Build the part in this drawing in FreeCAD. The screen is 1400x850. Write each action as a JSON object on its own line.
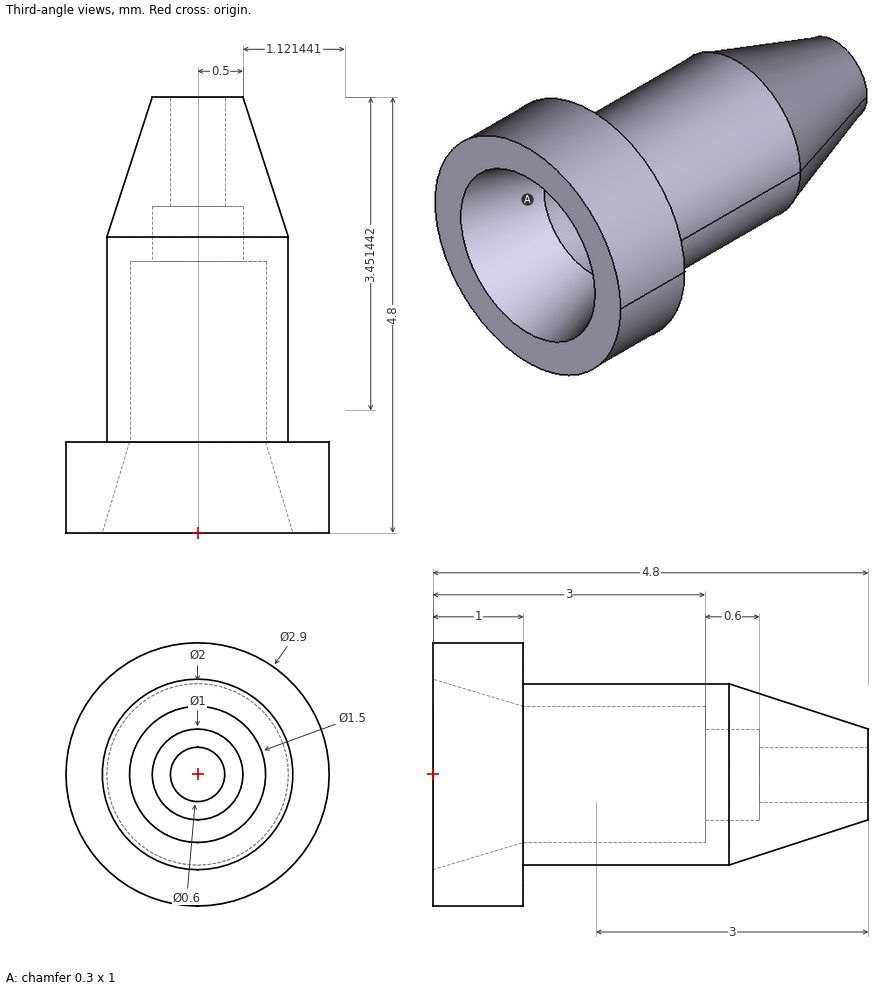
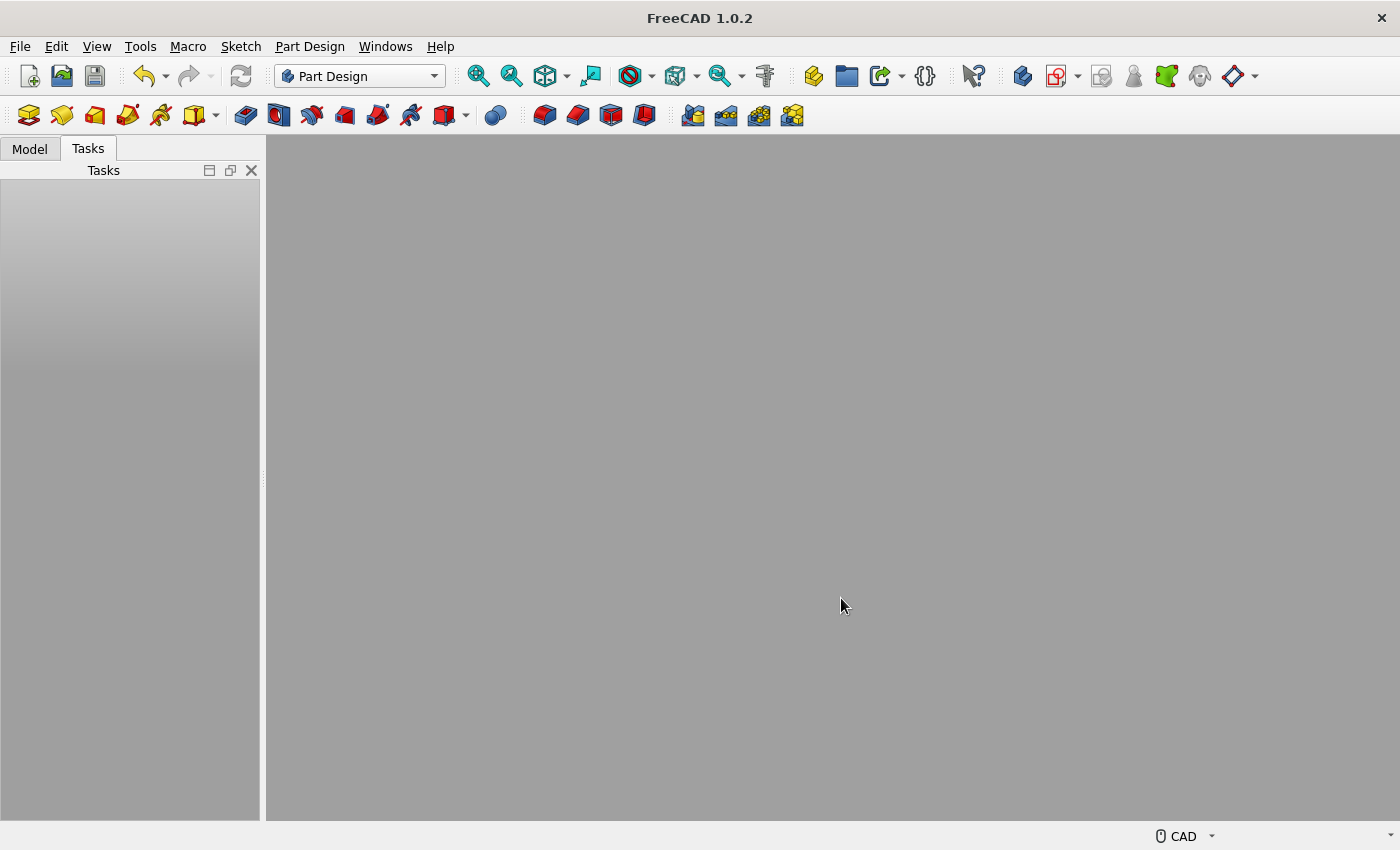
{"action": "left_click", "coordinate": [29, 76]}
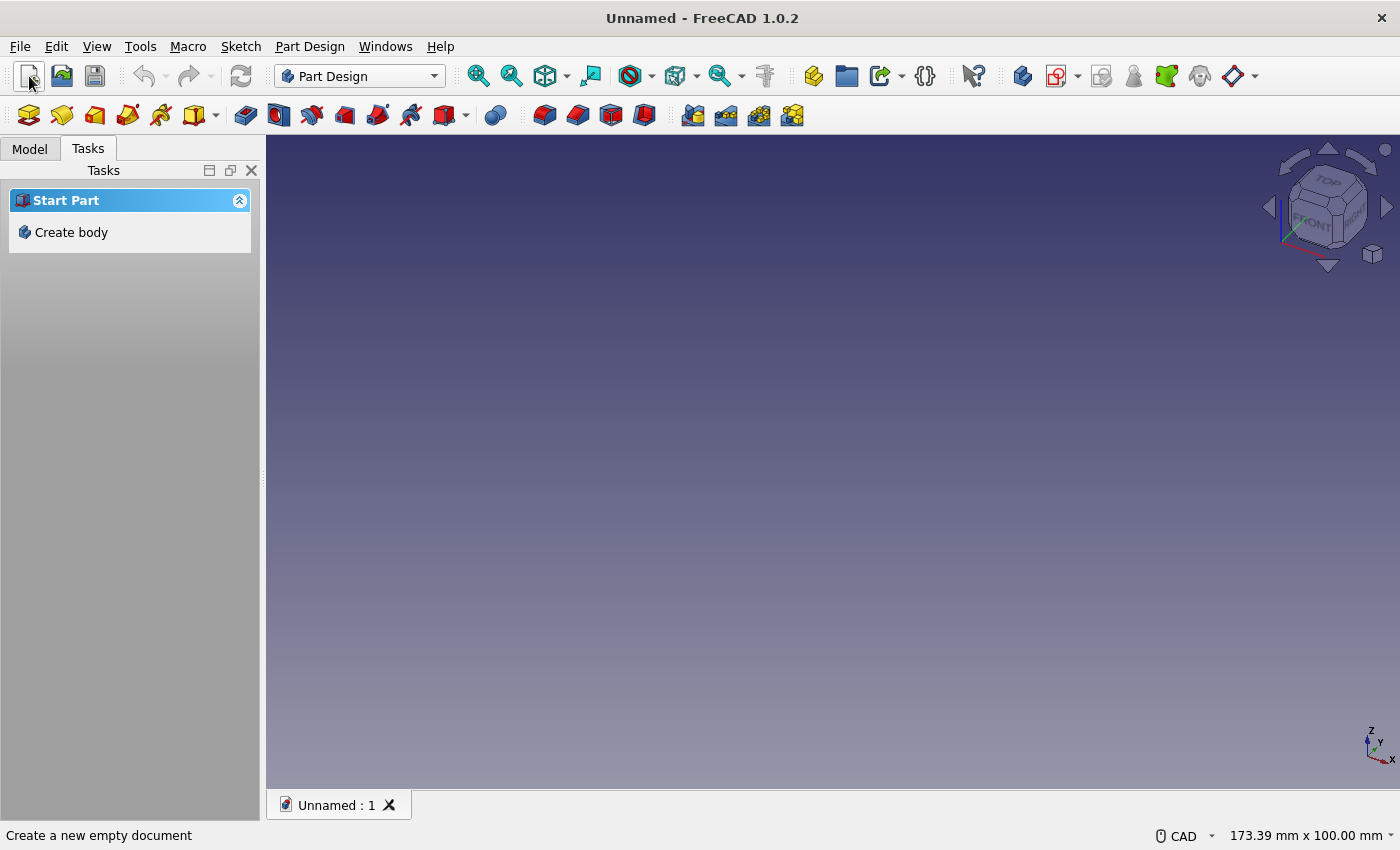
{"action": "left_click", "coordinate": [1056, 76]}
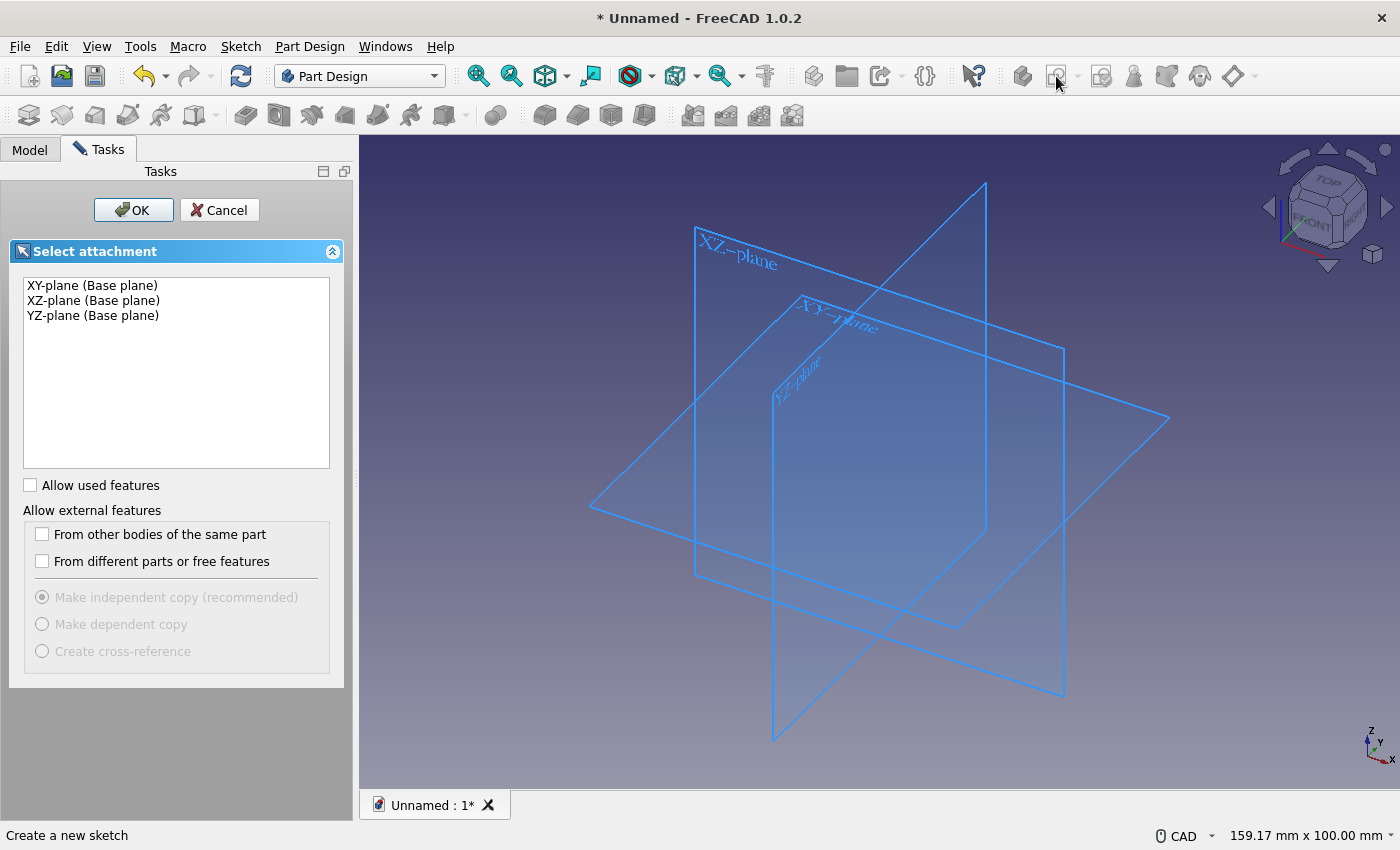
{"action": "left_click", "coordinate": [84, 300]}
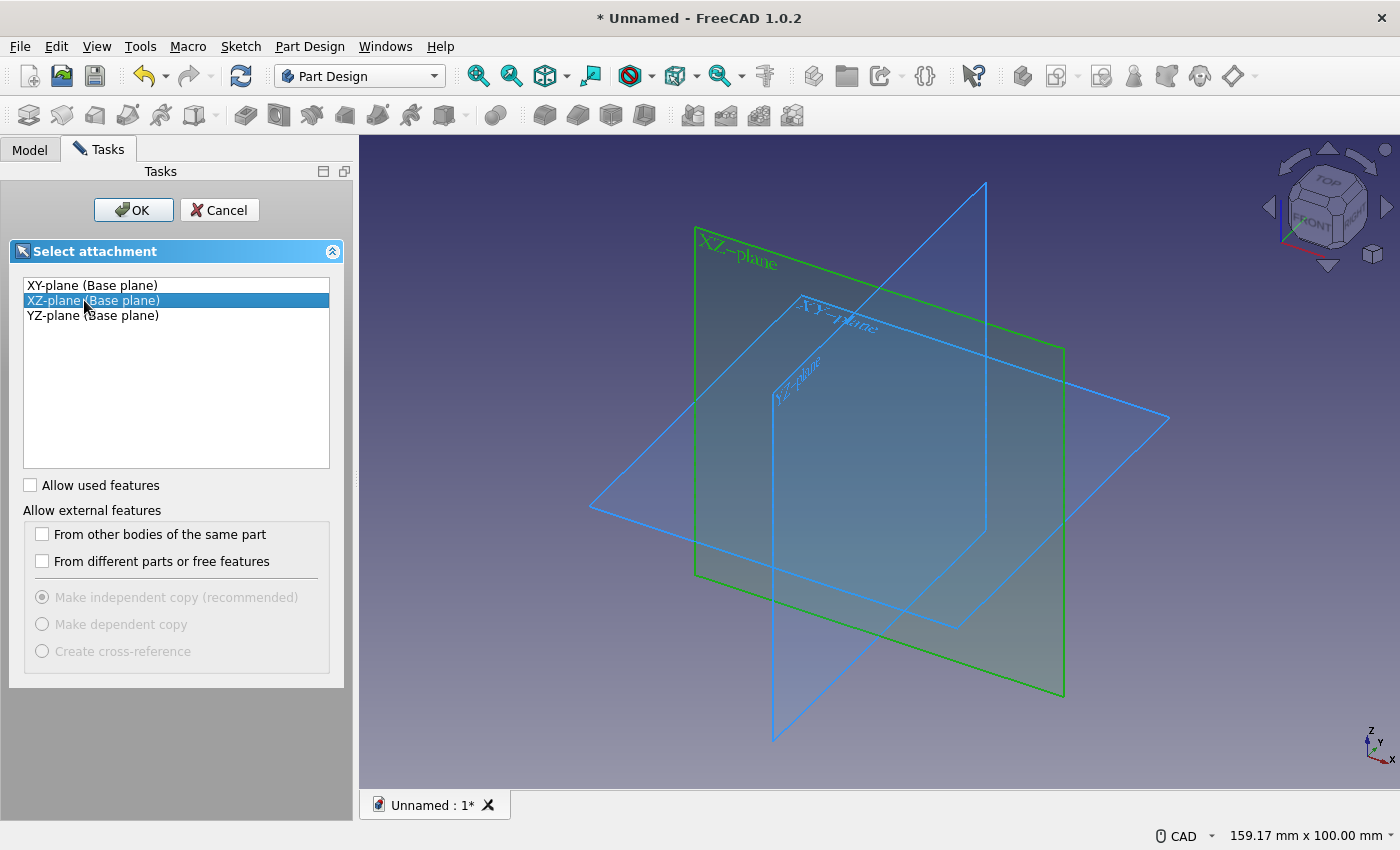
{"action": "left_click", "coordinate": [134, 210]}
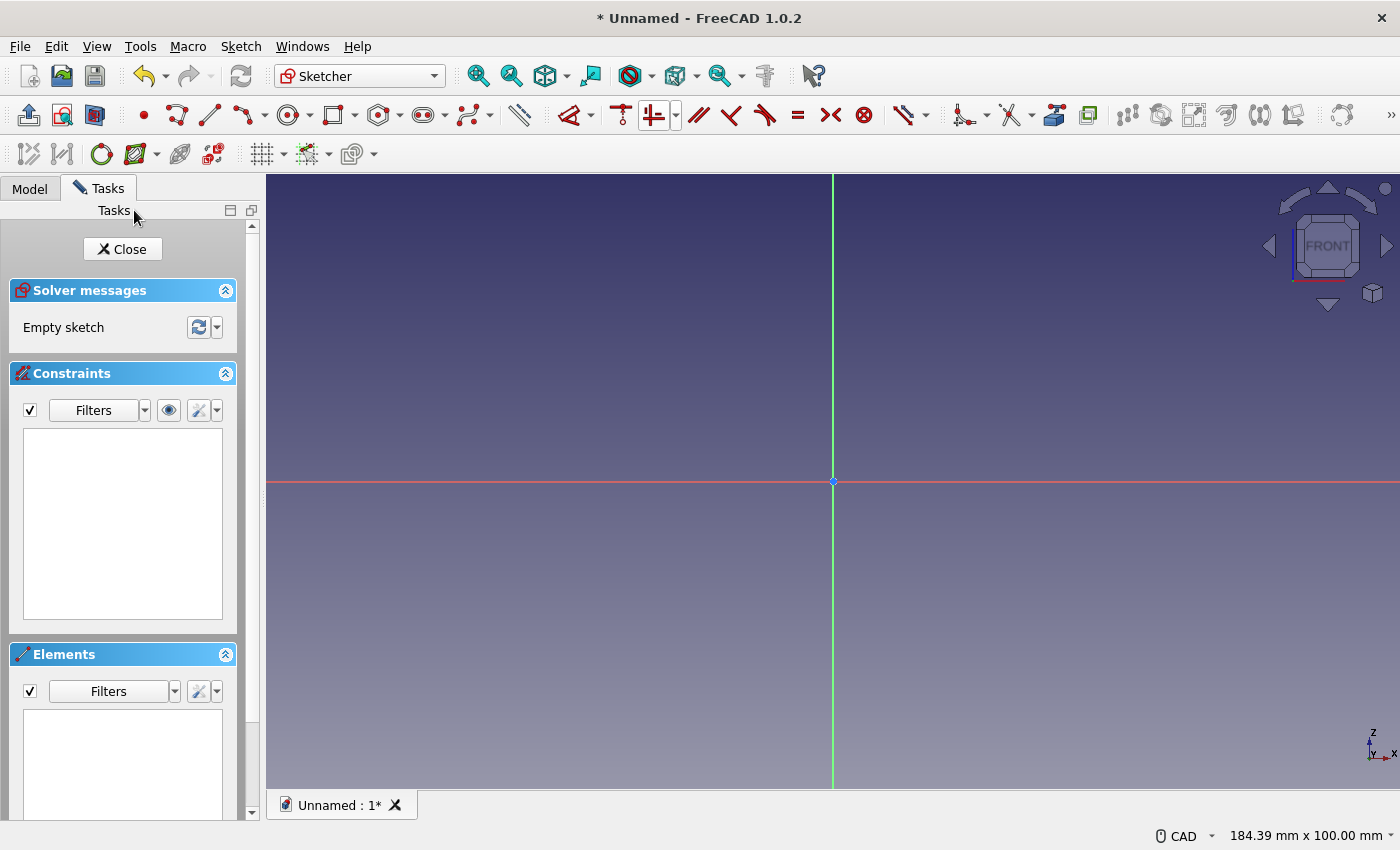
{"action": "scroll", "coordinate": [837, 481], "scroll_direction": "up", "scroll_amount": 15}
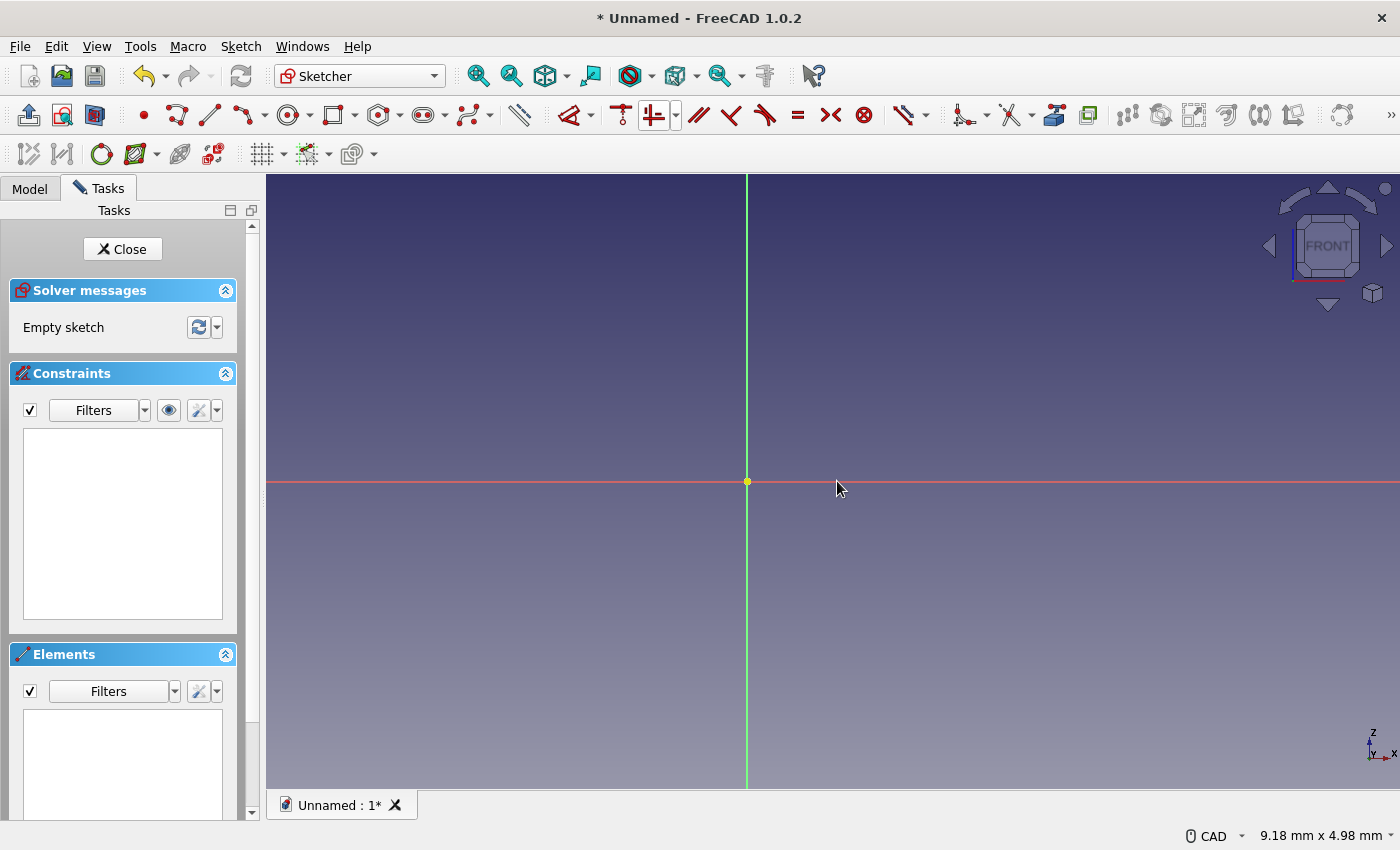
{"action": "scroll", "coordinate": [712, 482], "scroll_direction": "up", "scroll_amount": 2}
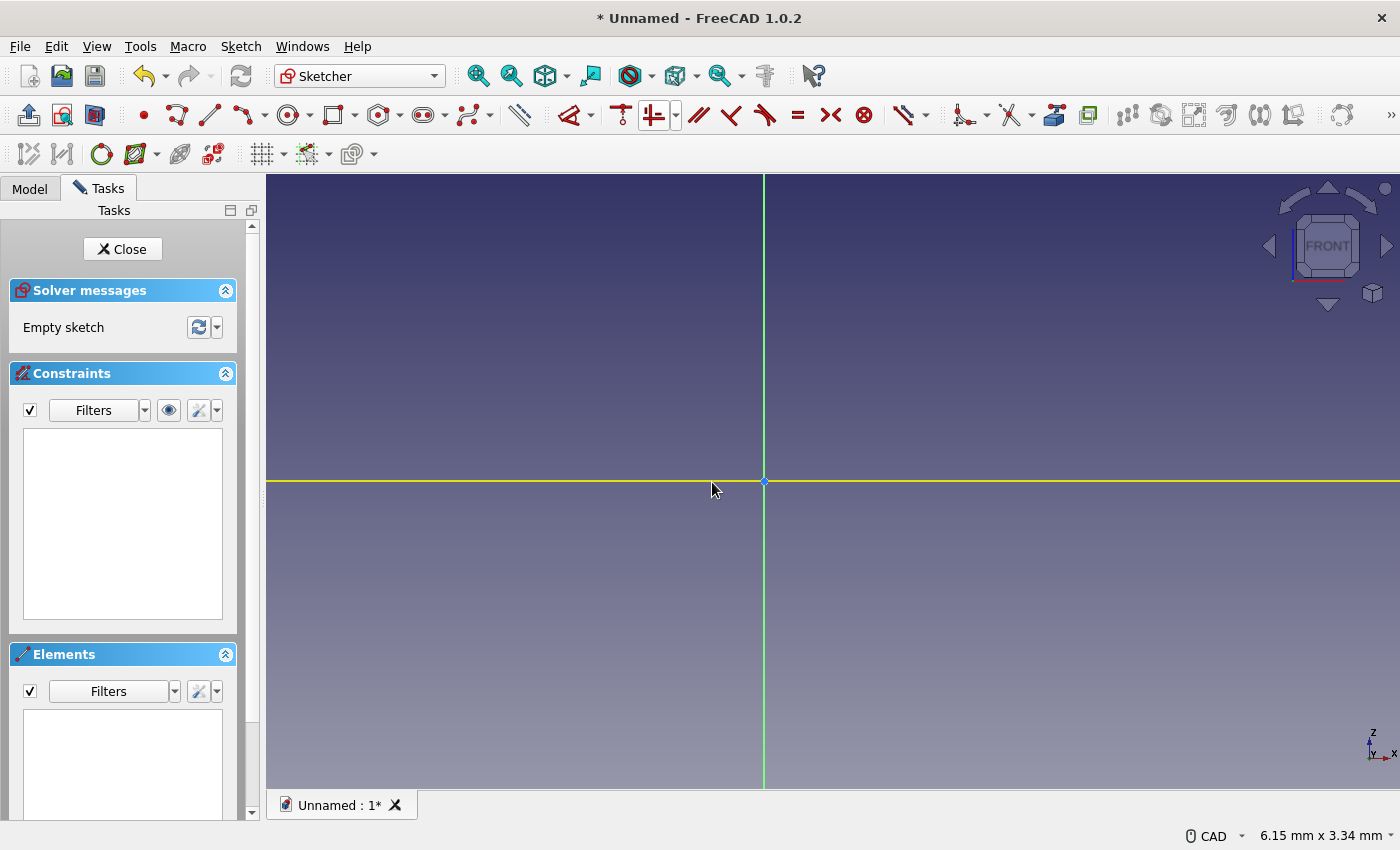
{"action": "left_click", "coordinate": [288, 116]}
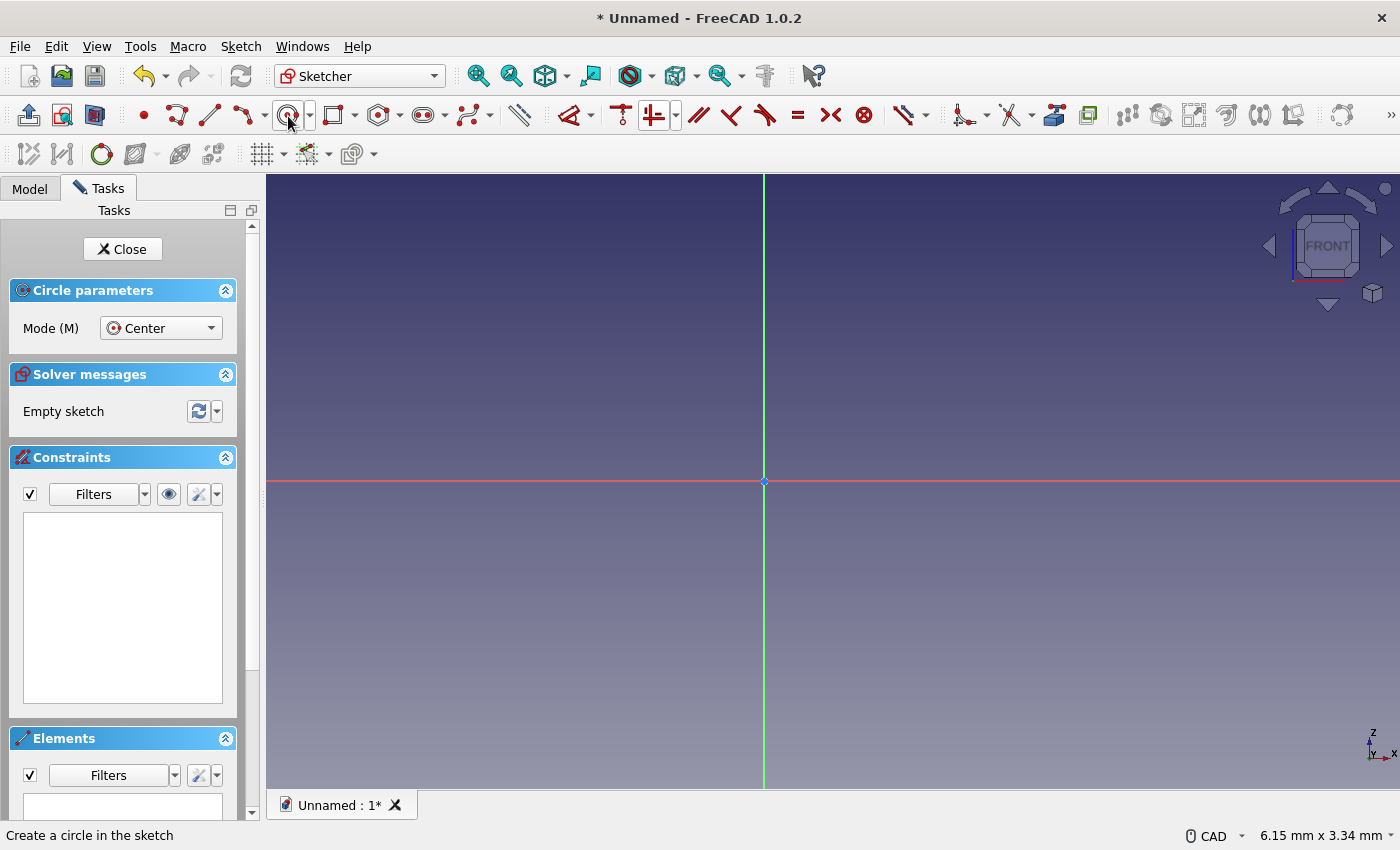
{"action": "left_click", "coordinate": [764, 481]}
{"action": "left_click", "coordinate": [894, 351]}
{"action": "key", "text": "Escape"}